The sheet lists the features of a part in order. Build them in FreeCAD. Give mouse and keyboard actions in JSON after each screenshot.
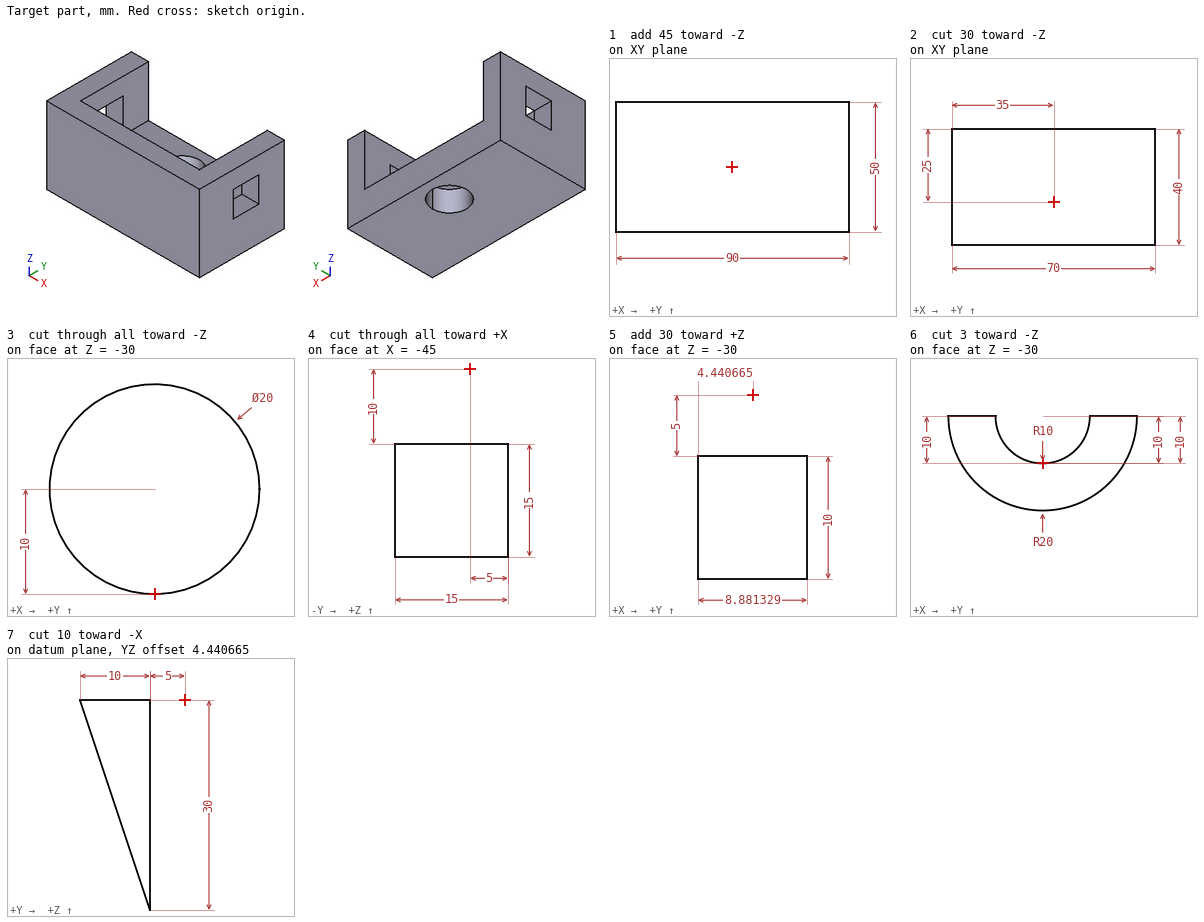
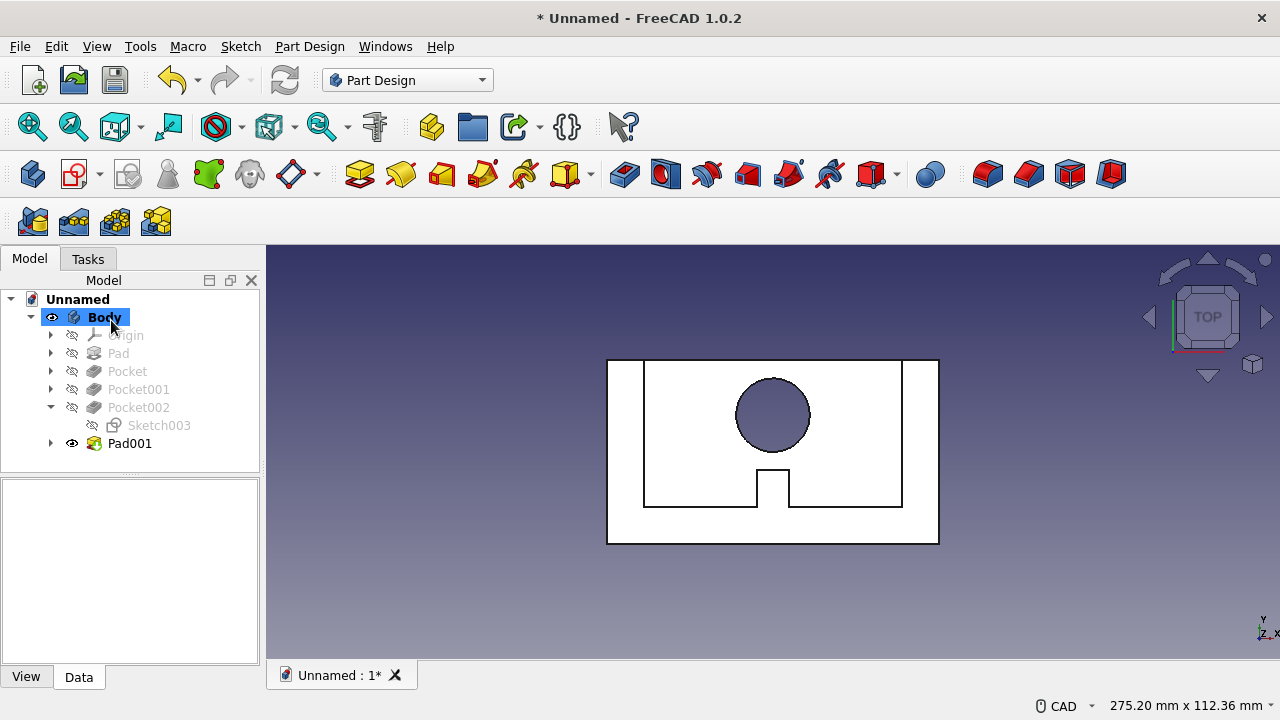
{"action": "key", "text": "v f"}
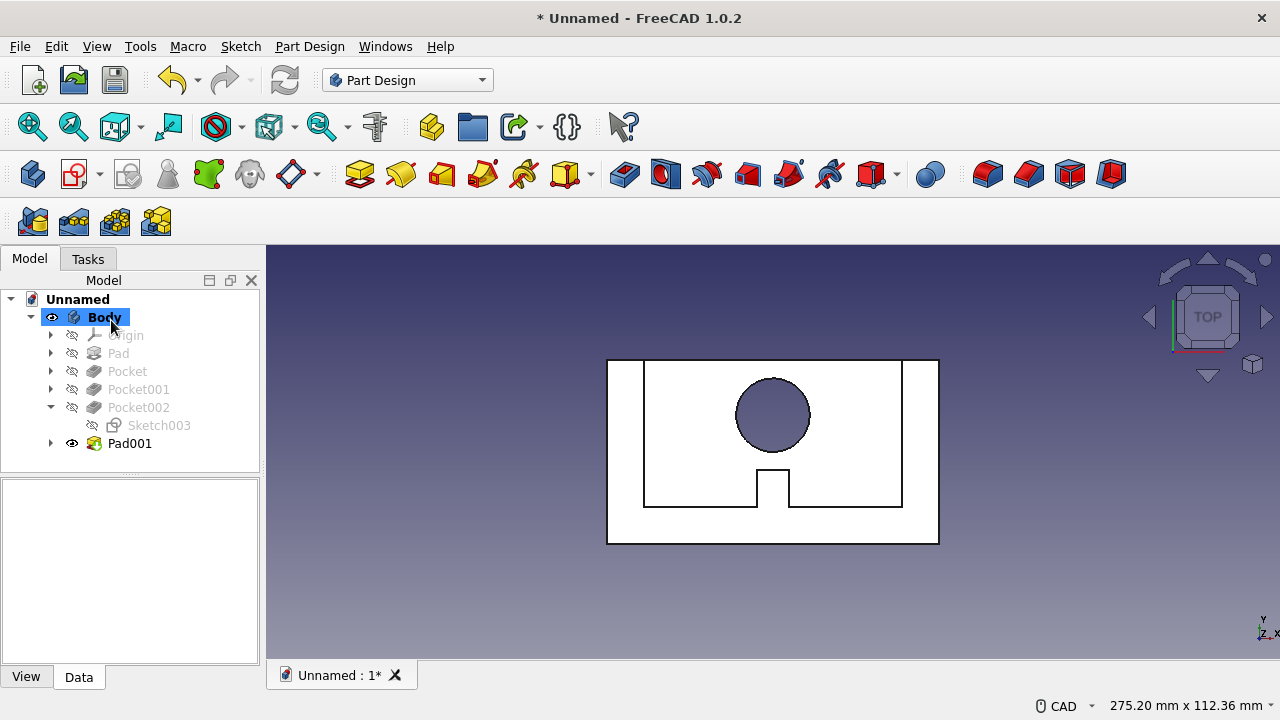
{"action": "left_click", "coordinate": [847, 454]}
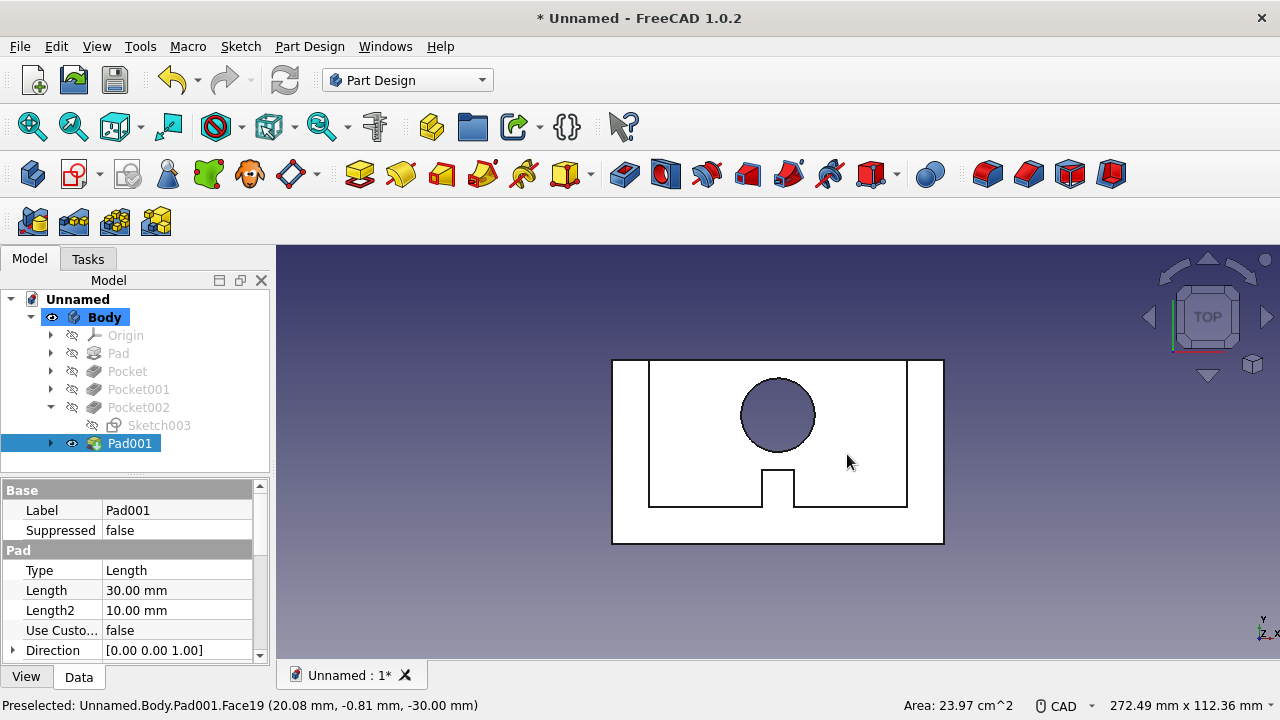
{"action": "left_click", "coordinate": [74, 174]}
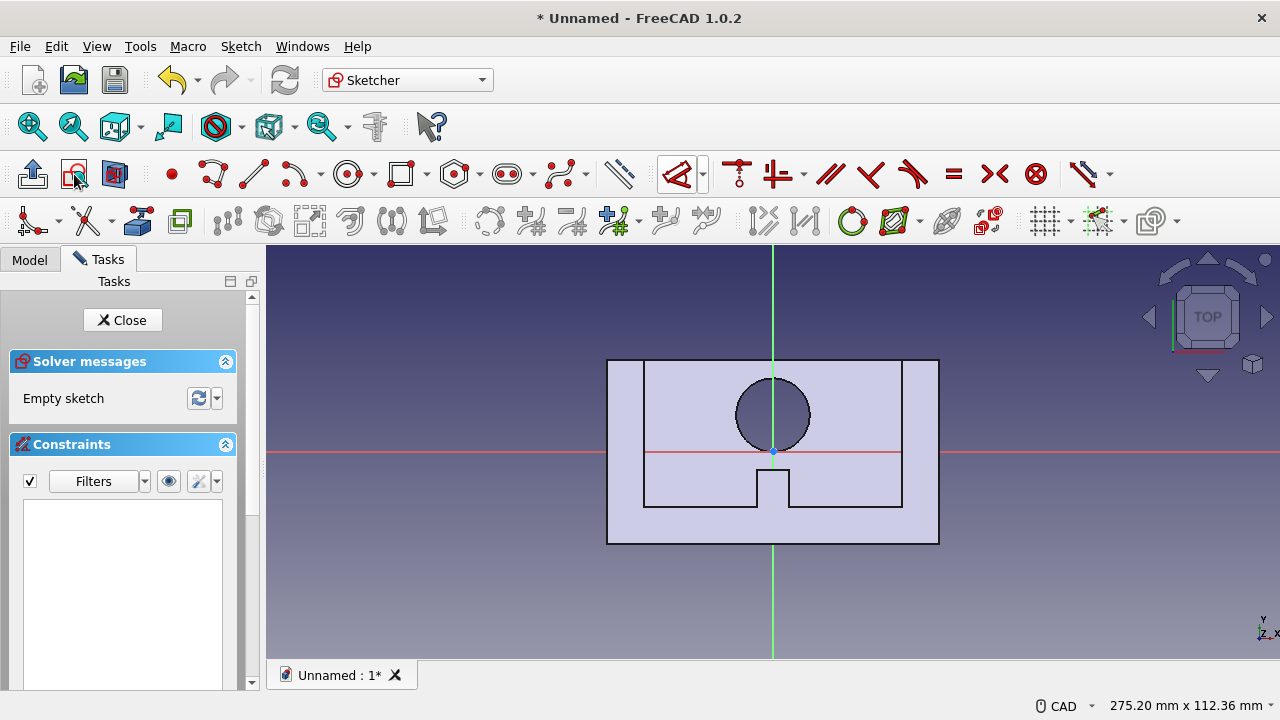
{"action": "scroll", "coordinate": [803, 452], "scroll_direction": "up", "scroll_amount": 6}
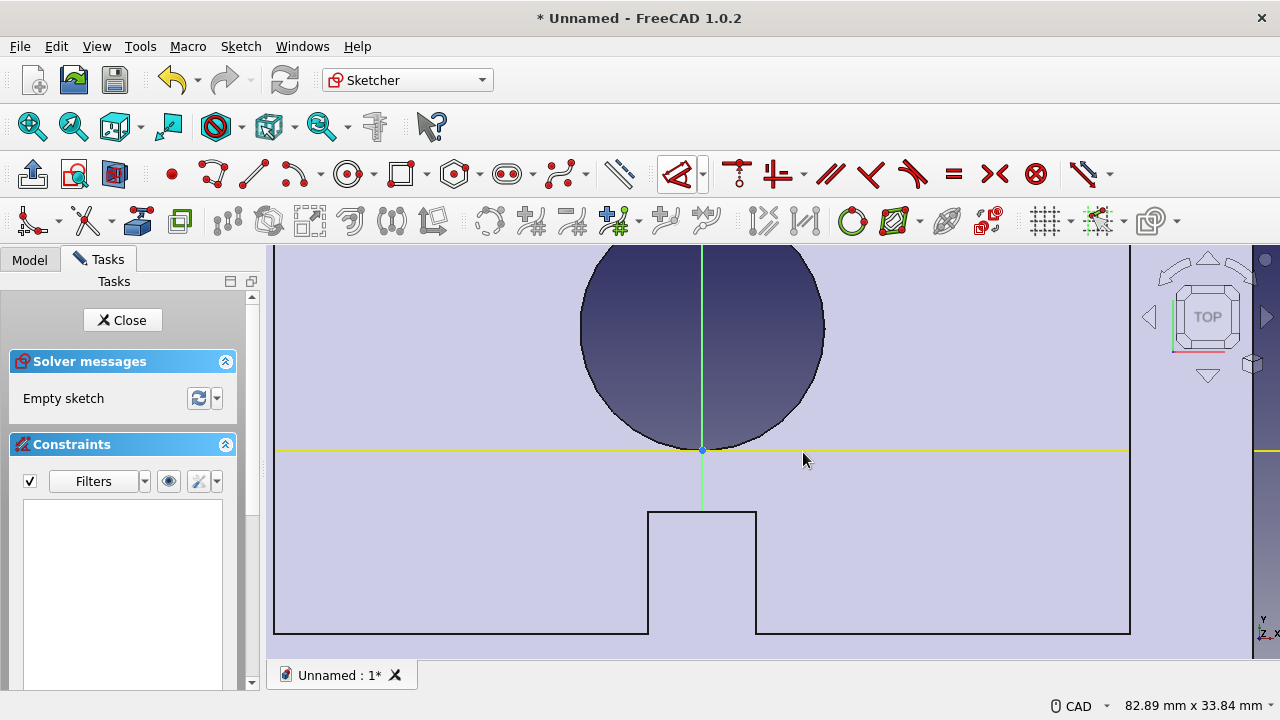
{"action": "key", "text": "g l"}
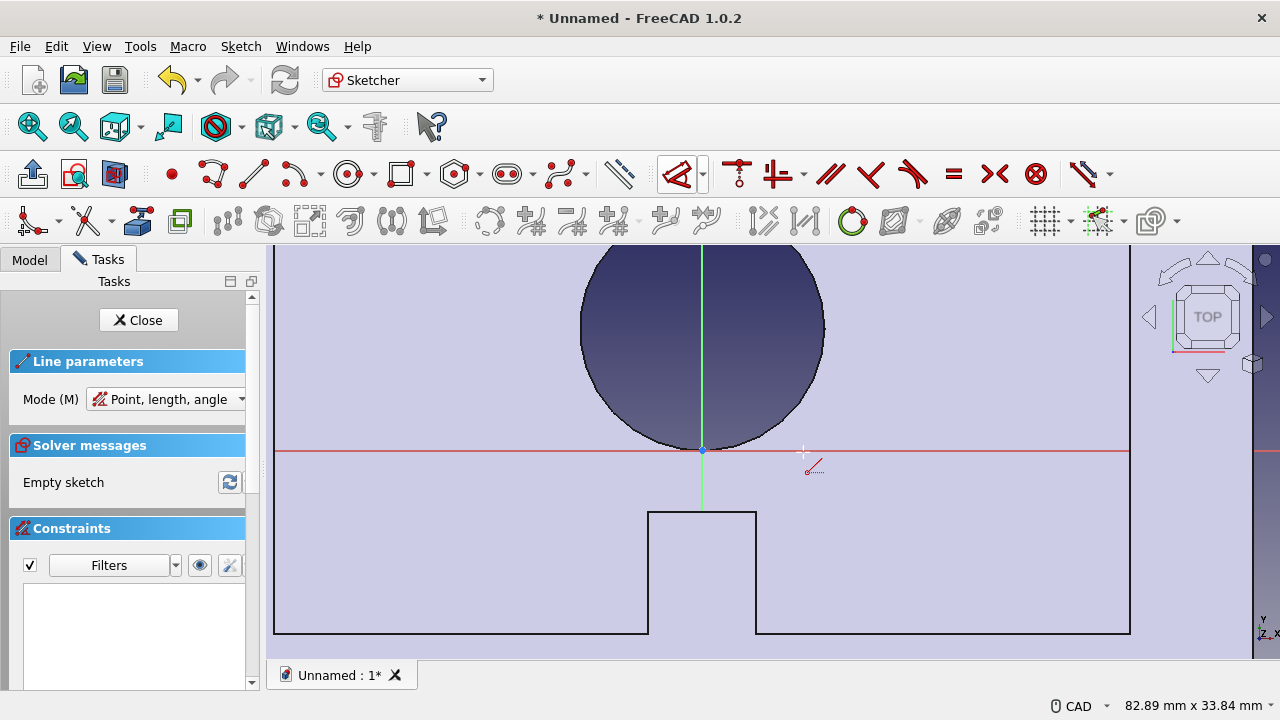
{"action": "left_click", "coordinate": [947, 329]}
{"action": "left_click", "coordinate": [824, 329]}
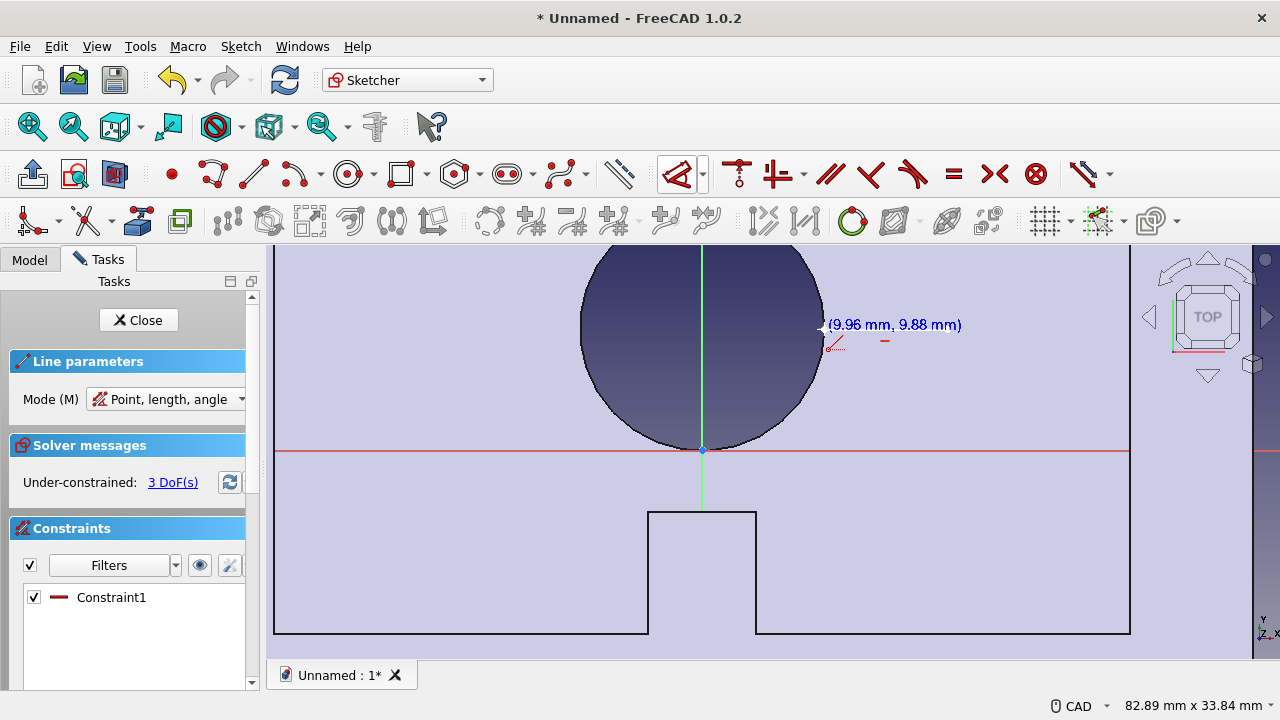
{"action": "left_click", "coordinate": [580, 329]}
{"action": "left_click", "coordinate": [458, 329]}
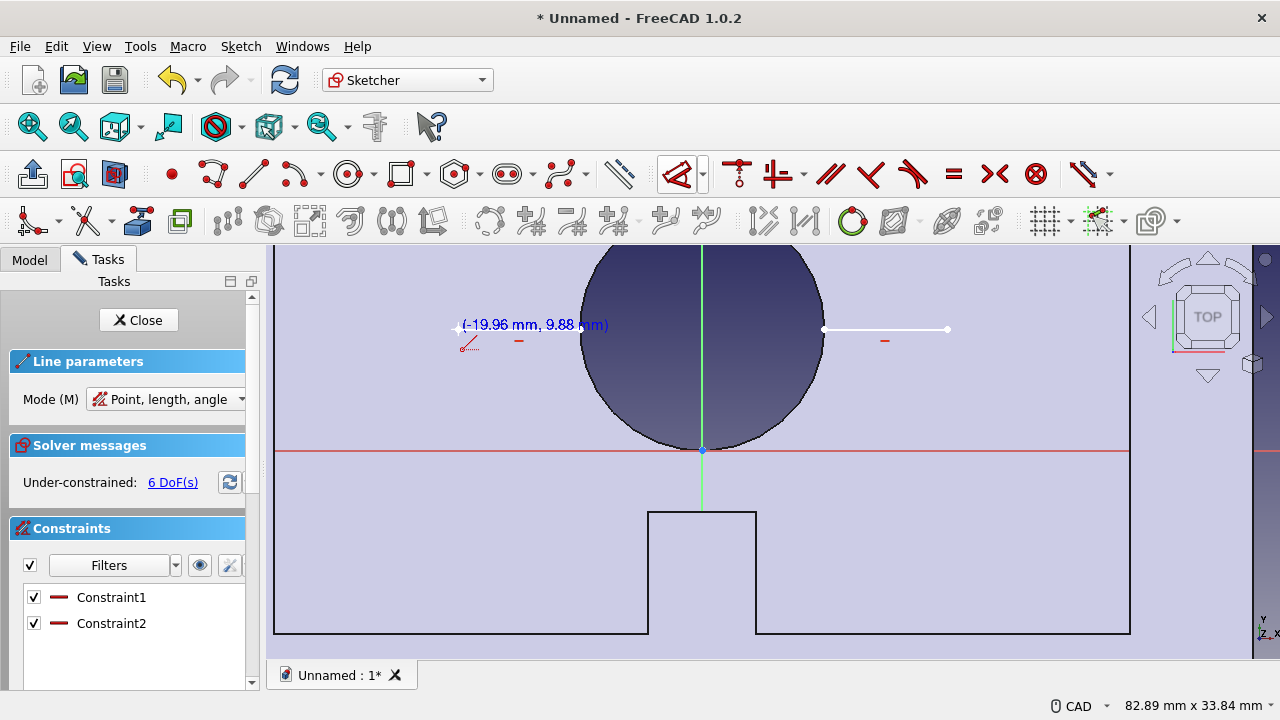
{"action": "key", "text": "g 3 a"}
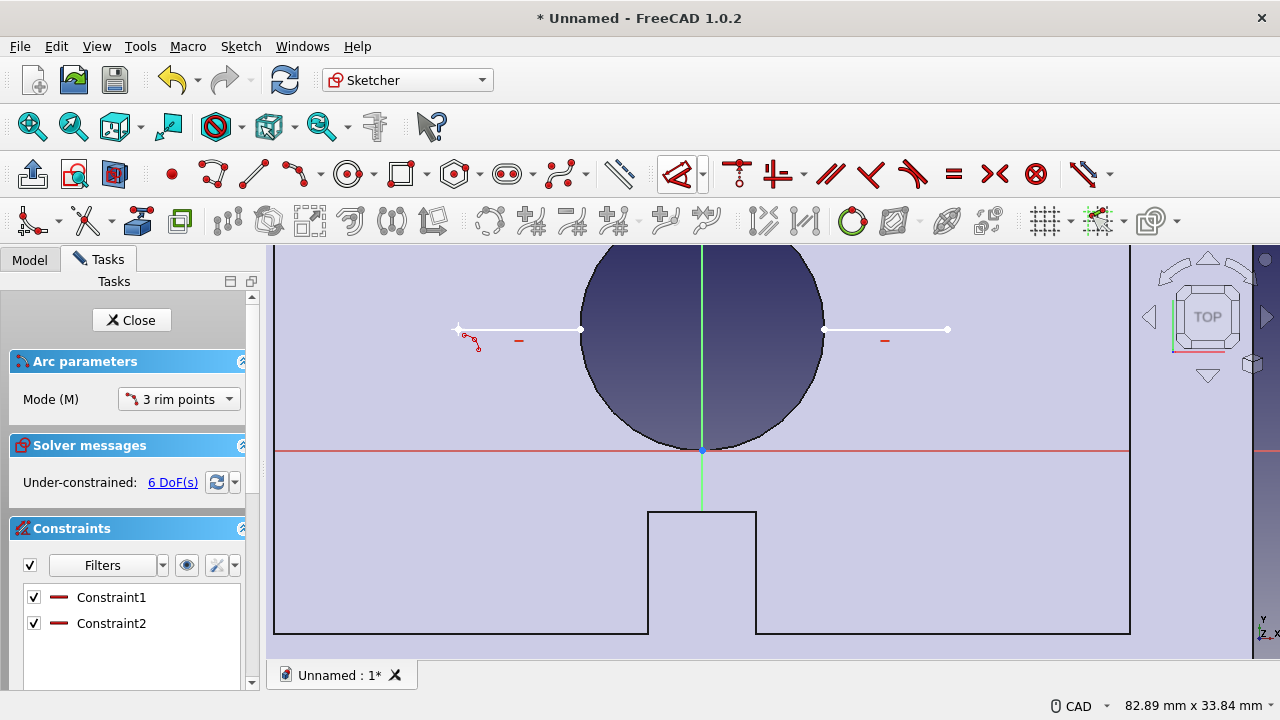
{"action": "left_click", "coordinate": [824, 330]}
{"action": "left_click", "coordinate": [580, 330]}
{"action": "left_click", "coordinate": [630, 427]}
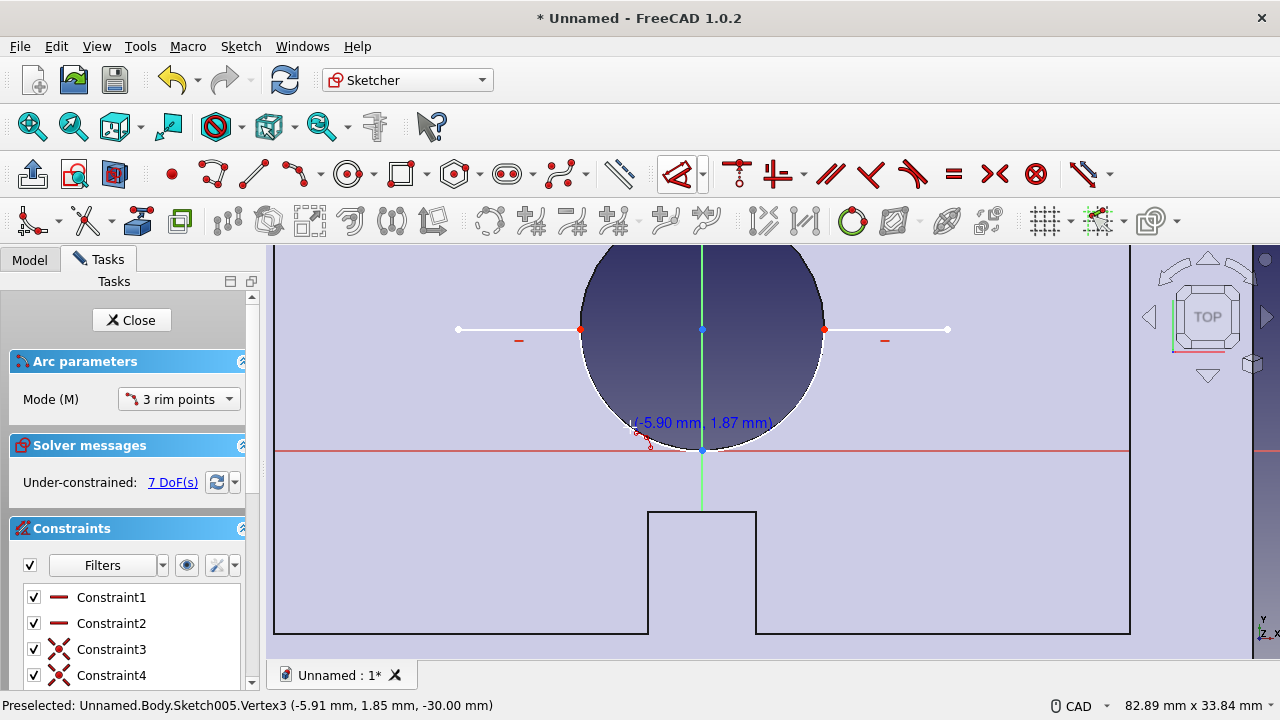
{"action": "left_click", "coordinate": [458, 330]}
{"action": "left_click", "coordinate": [947, 330]}
{"action": "left_click", "coordinate": [627, 561]}
{"action": "key", "text": "Escape"}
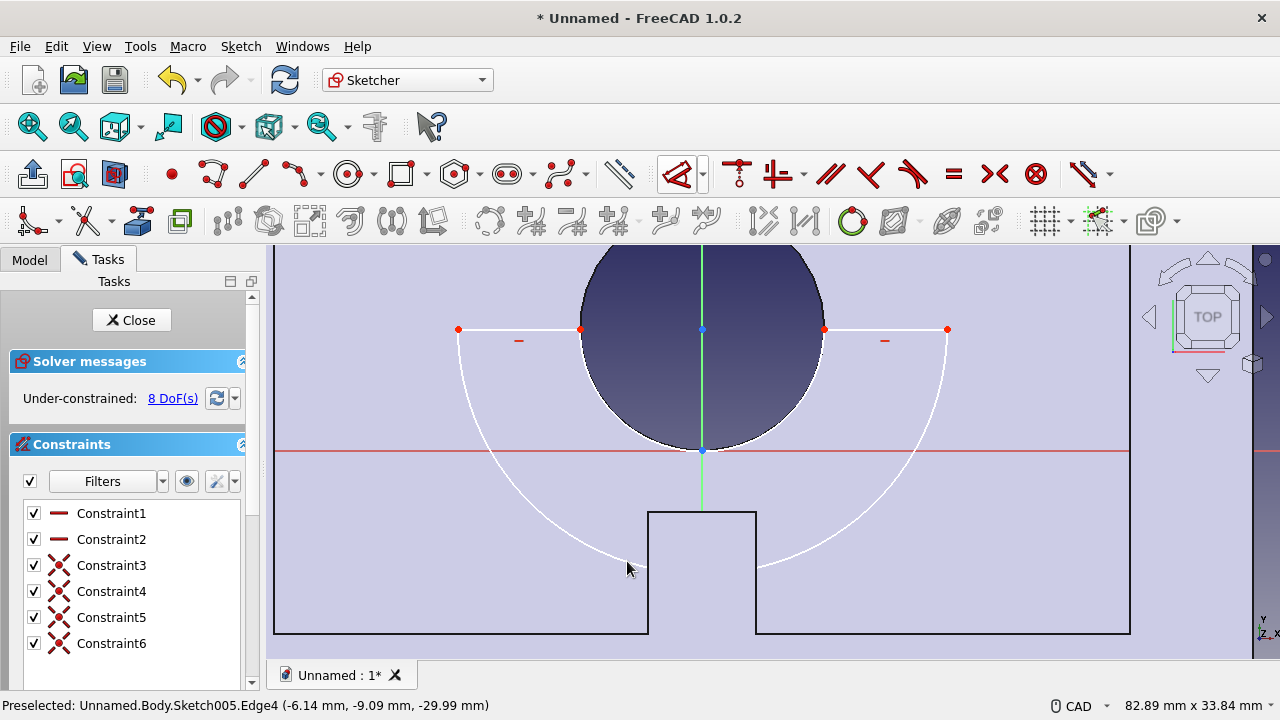
{"action": "left_click", "coordinate": [630, 428]}